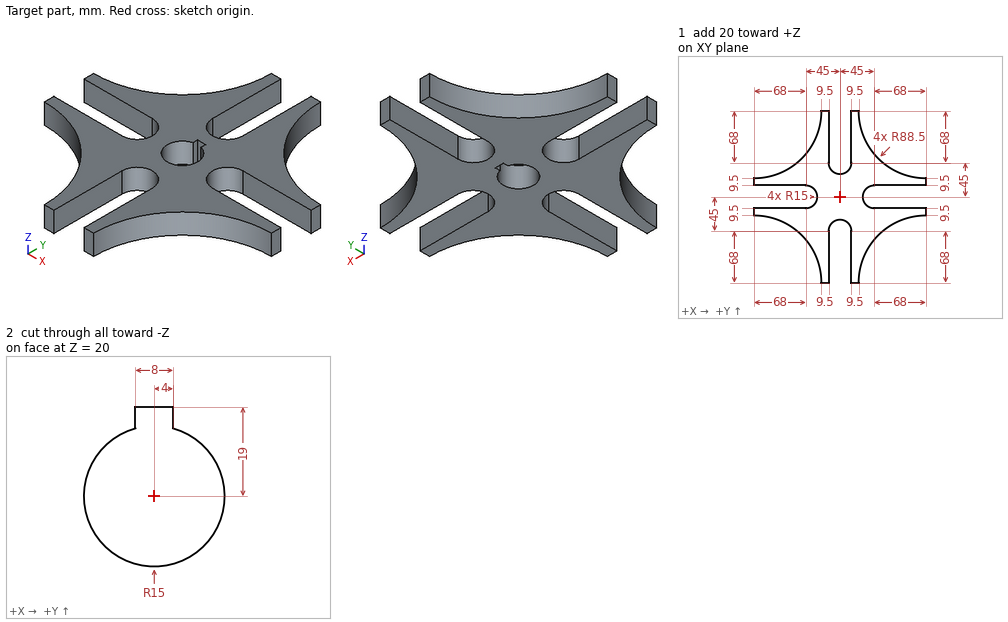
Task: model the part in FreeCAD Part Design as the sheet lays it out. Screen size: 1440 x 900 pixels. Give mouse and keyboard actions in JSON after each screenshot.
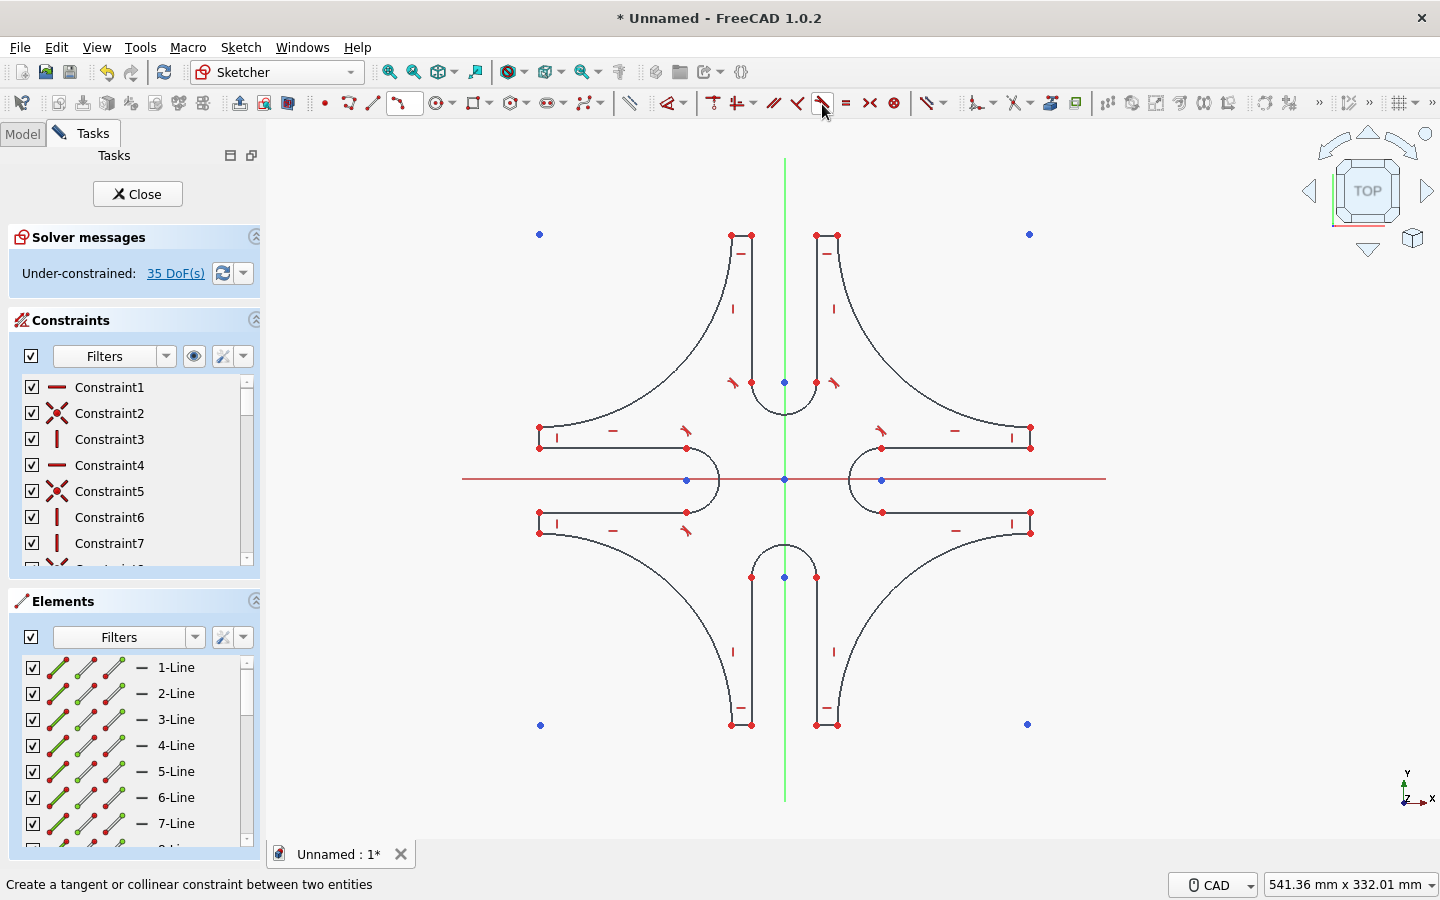
{"action": "left_click", "coordinate": [752, 681]}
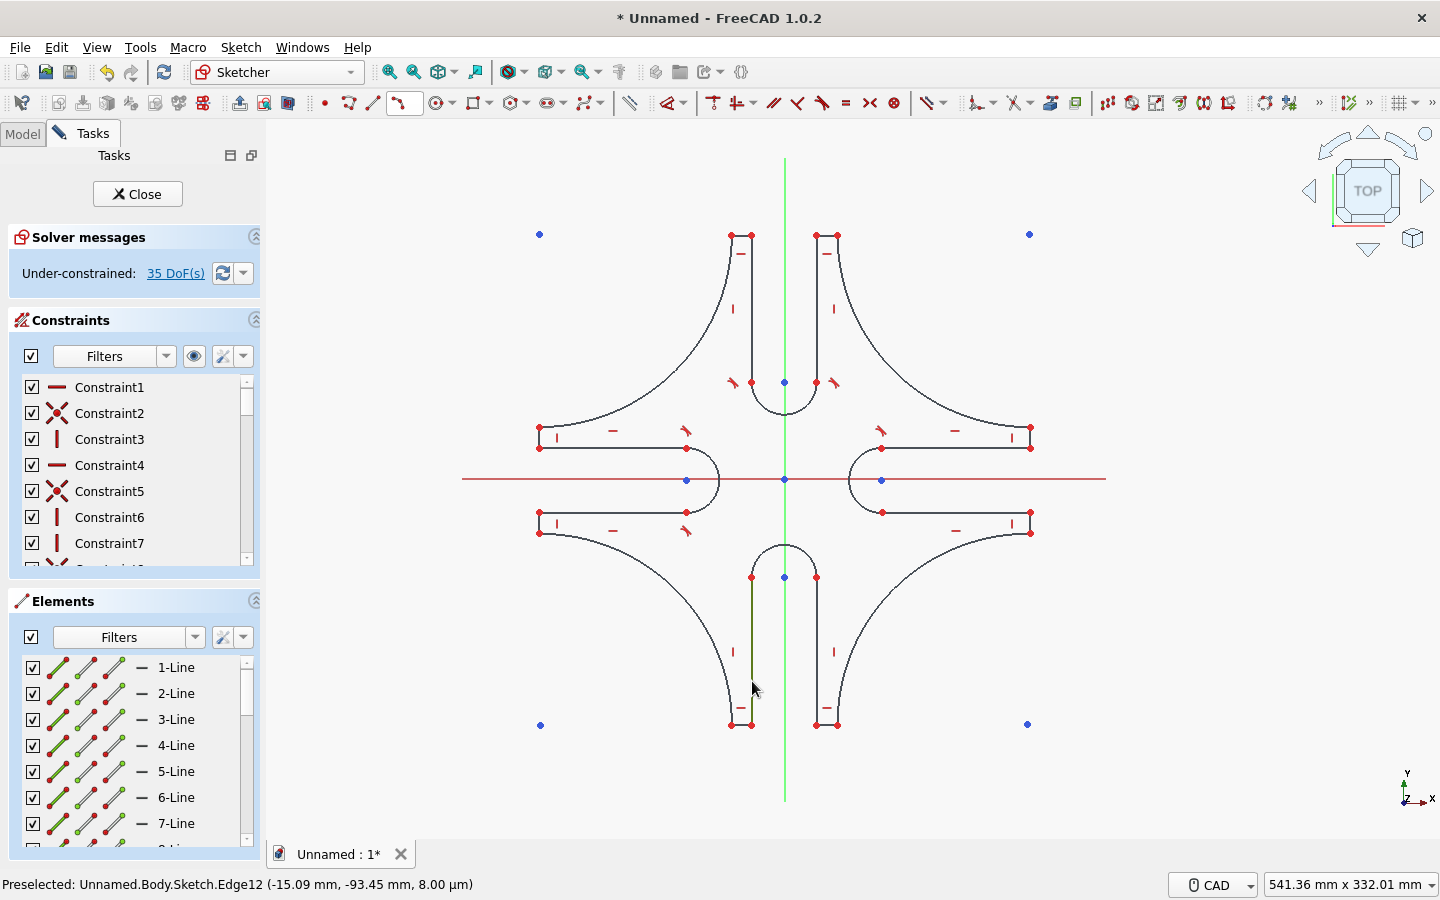
{"action": "left_click", "coordinate": [803, 551]}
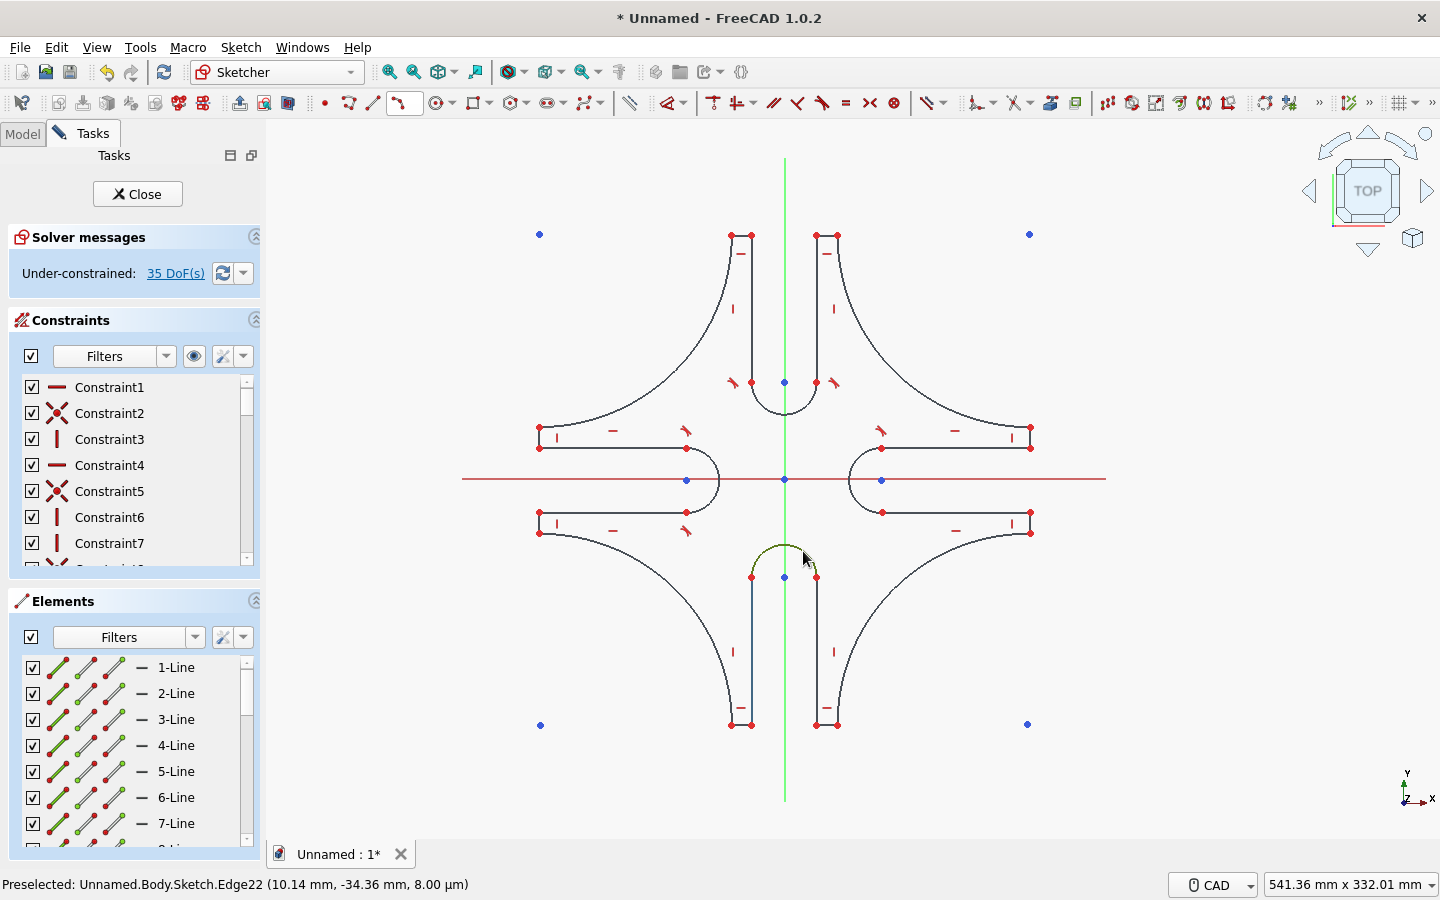
{"action": "left_click", "coordinate": [822, 104]}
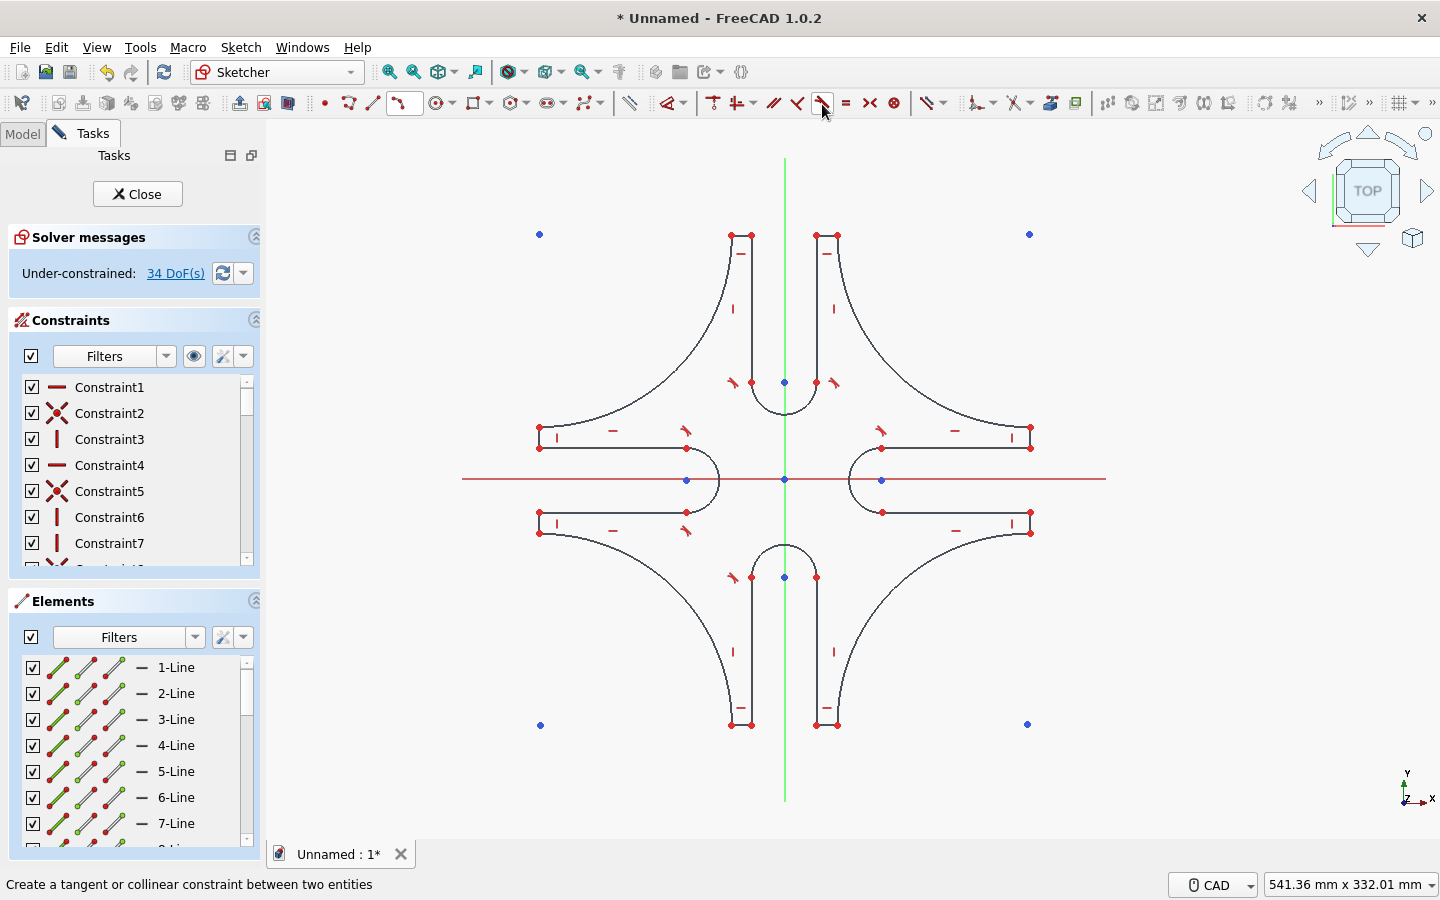
{"action": "left_click", "coordinate": [817, 622]}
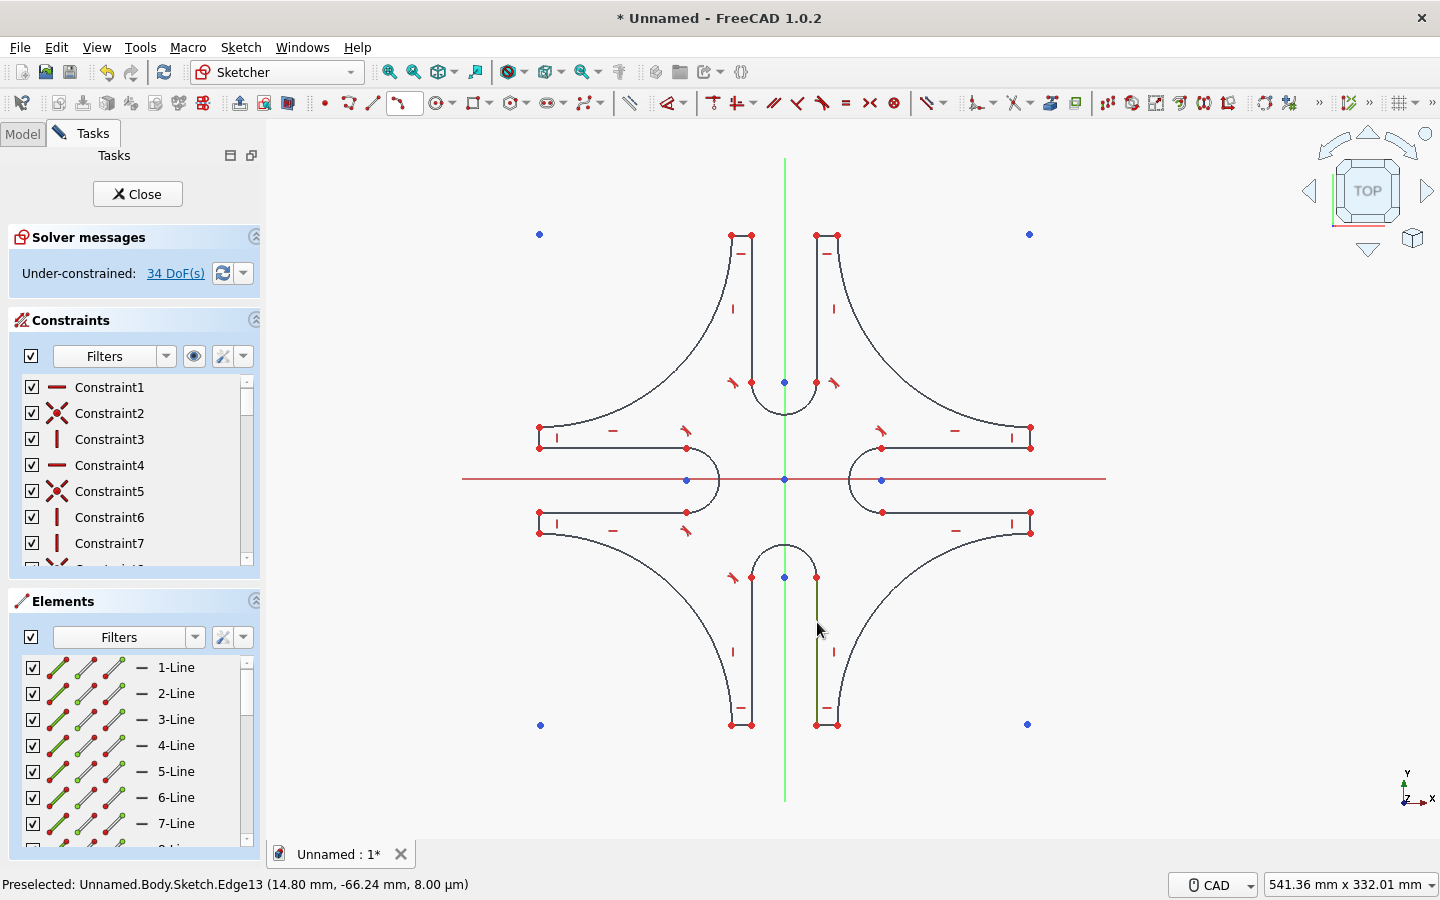
{"action": "left_click", "coordinate": [803, 551]}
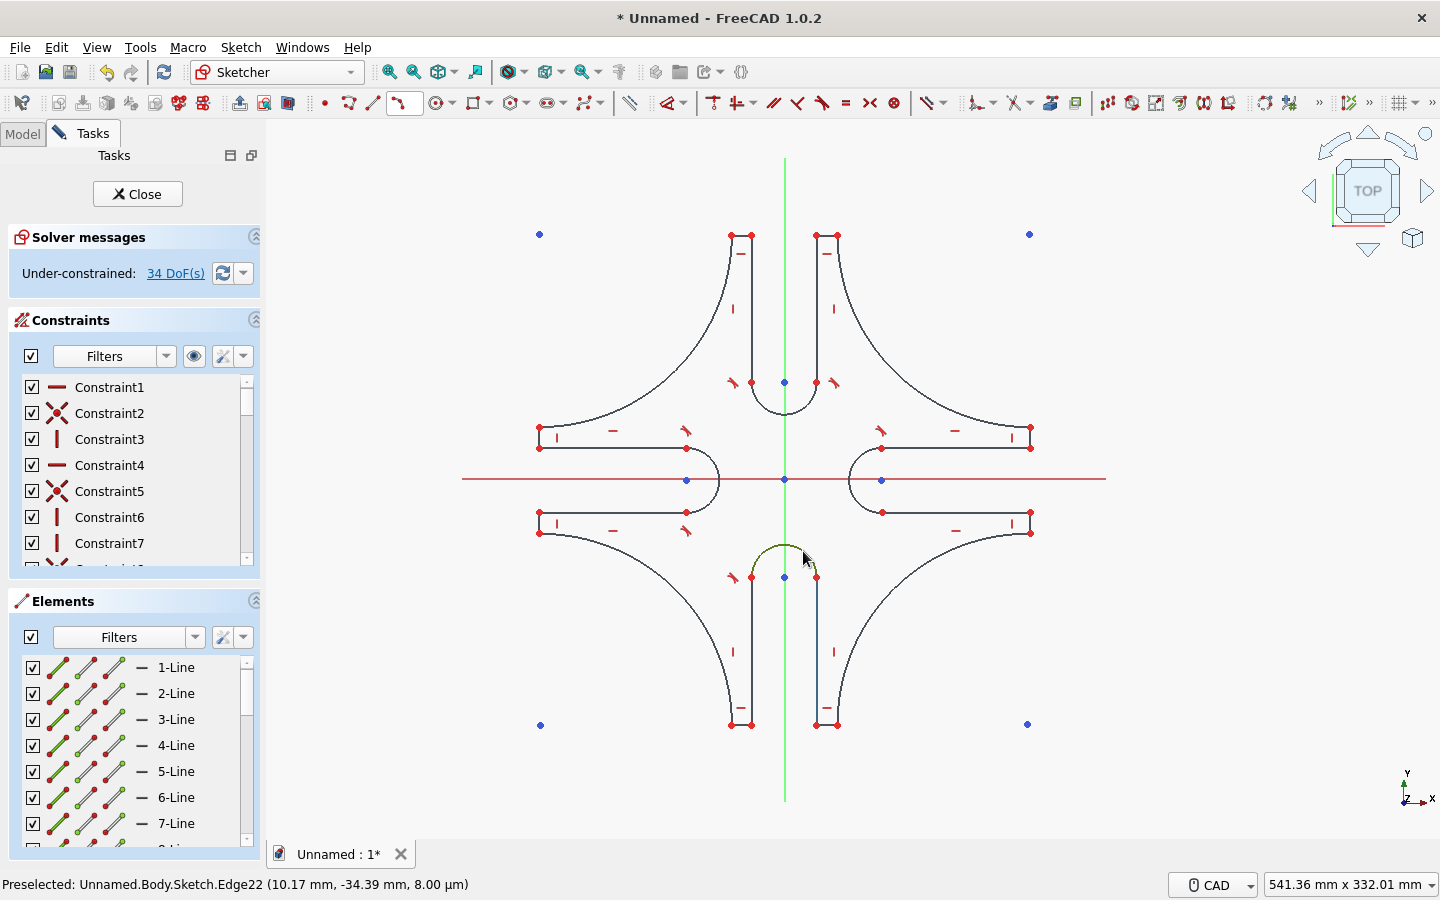
{"action": "left_click", "coordinate": [822, 104]}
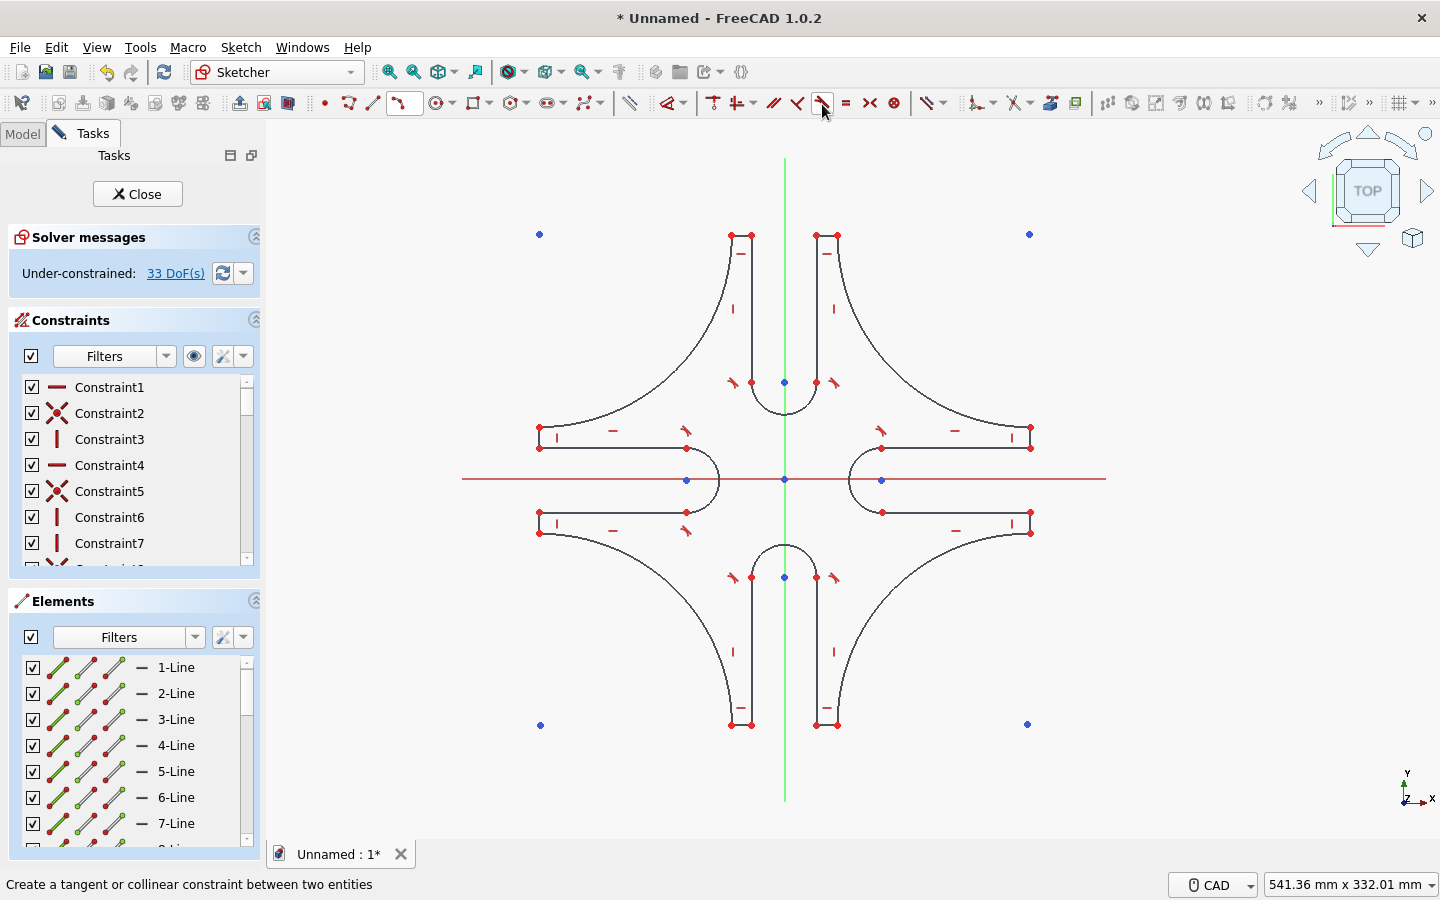
{"action": "left_click", "coordinate": [986, 513]}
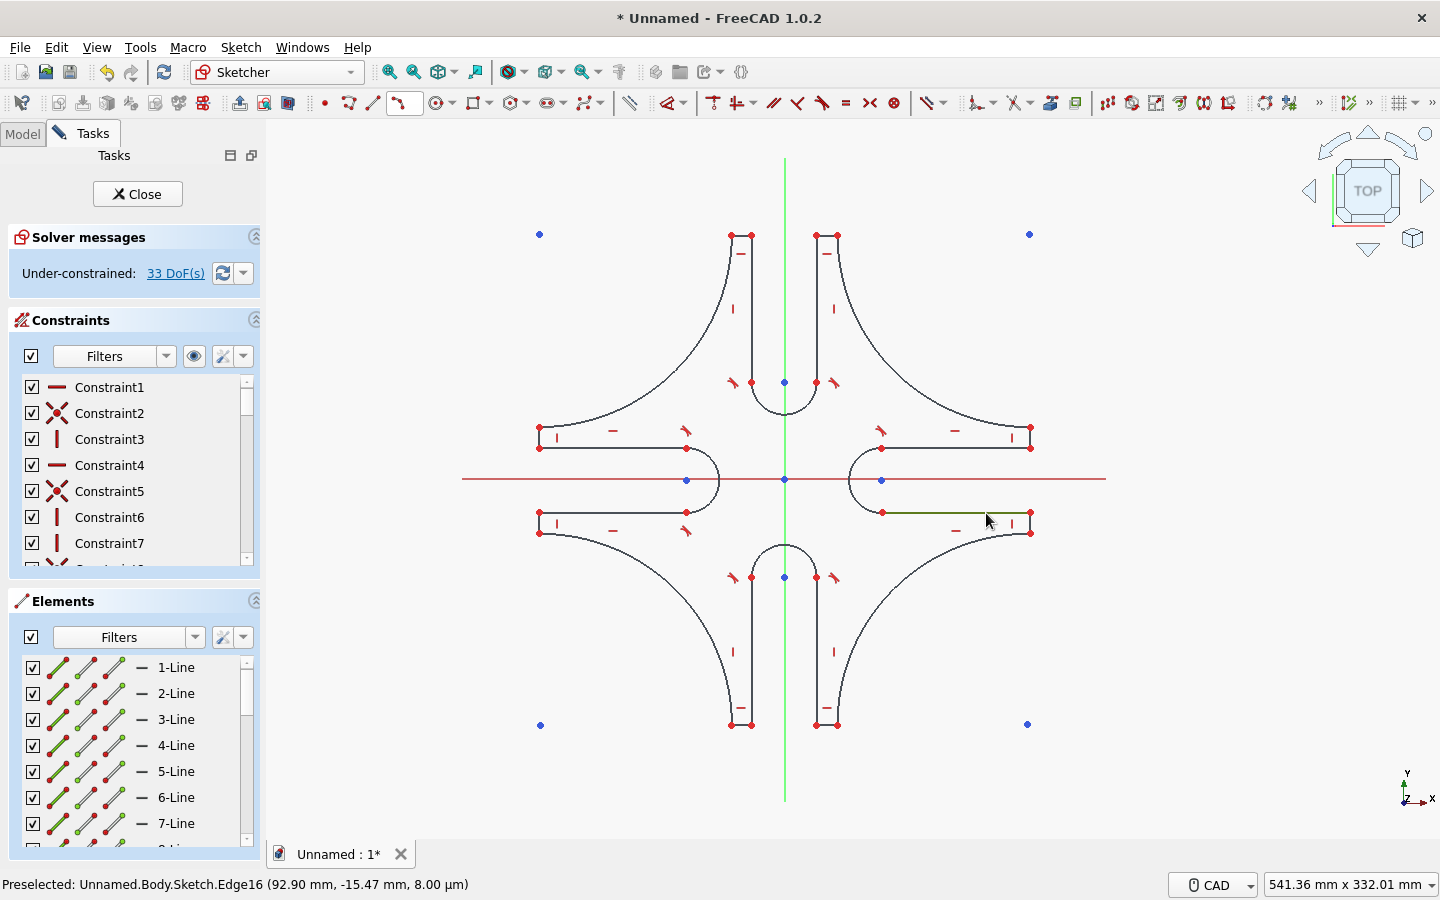
{"action": "left_click", "coordinate": [855, 462]}